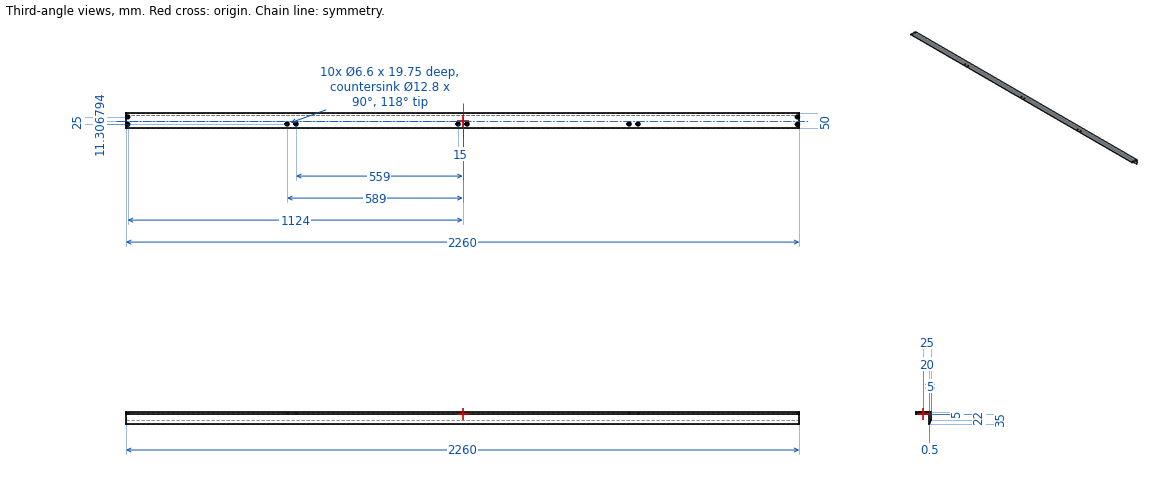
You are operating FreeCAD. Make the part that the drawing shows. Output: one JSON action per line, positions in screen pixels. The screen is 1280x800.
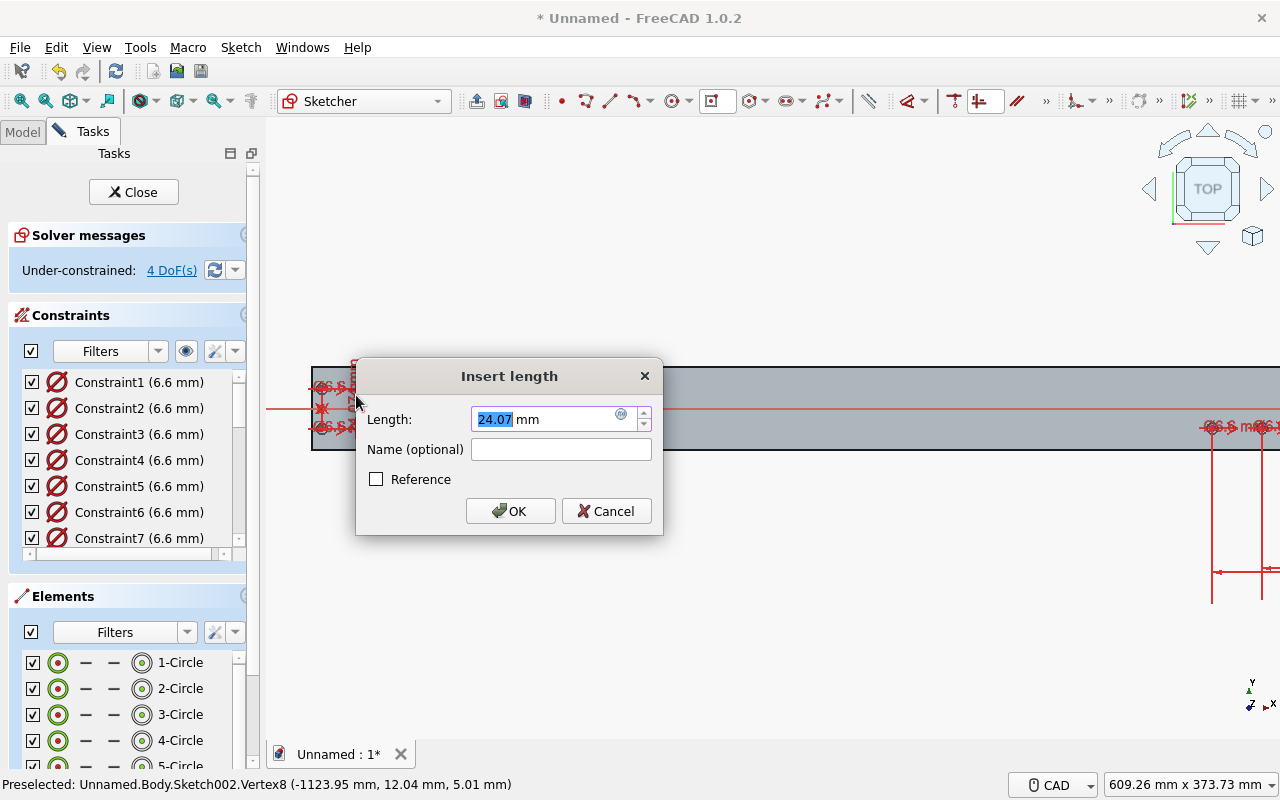
{"action": "type", "text": "25"}
{"action": "key", "text": "Return"}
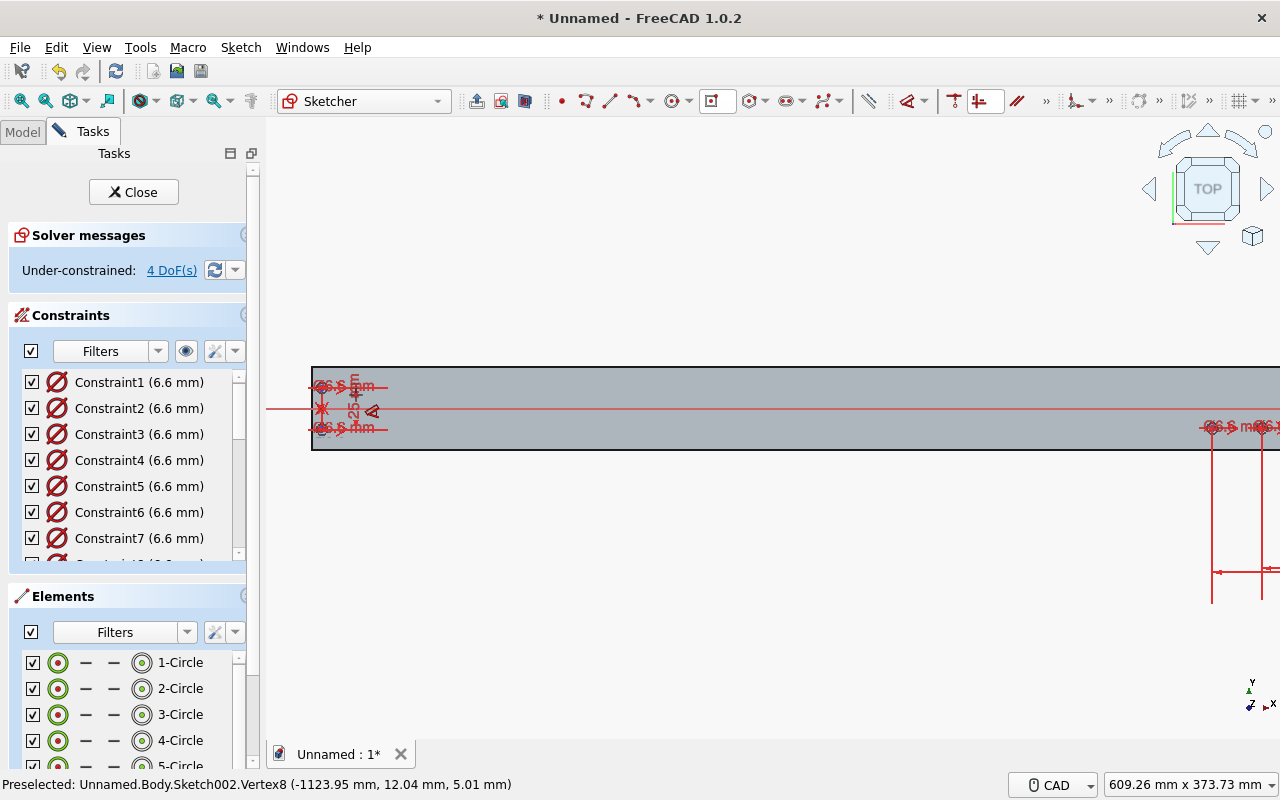
{"action": "scroll", "coordinate": [410, 432], "scroll_direction": "down", "scroll_amount": 9}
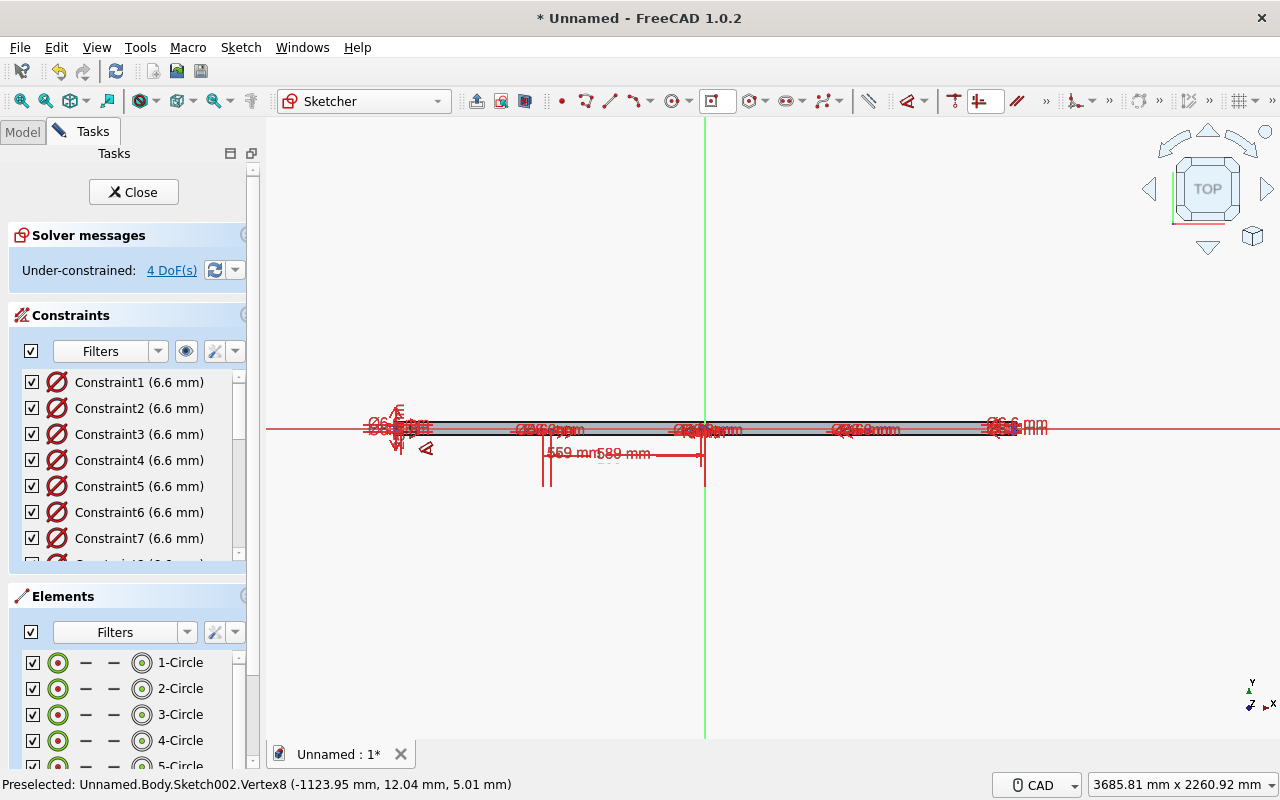
{"action": "scroll", "coordinate": [396, 432], "scroll_direction": "up", "scroll_amount": 3}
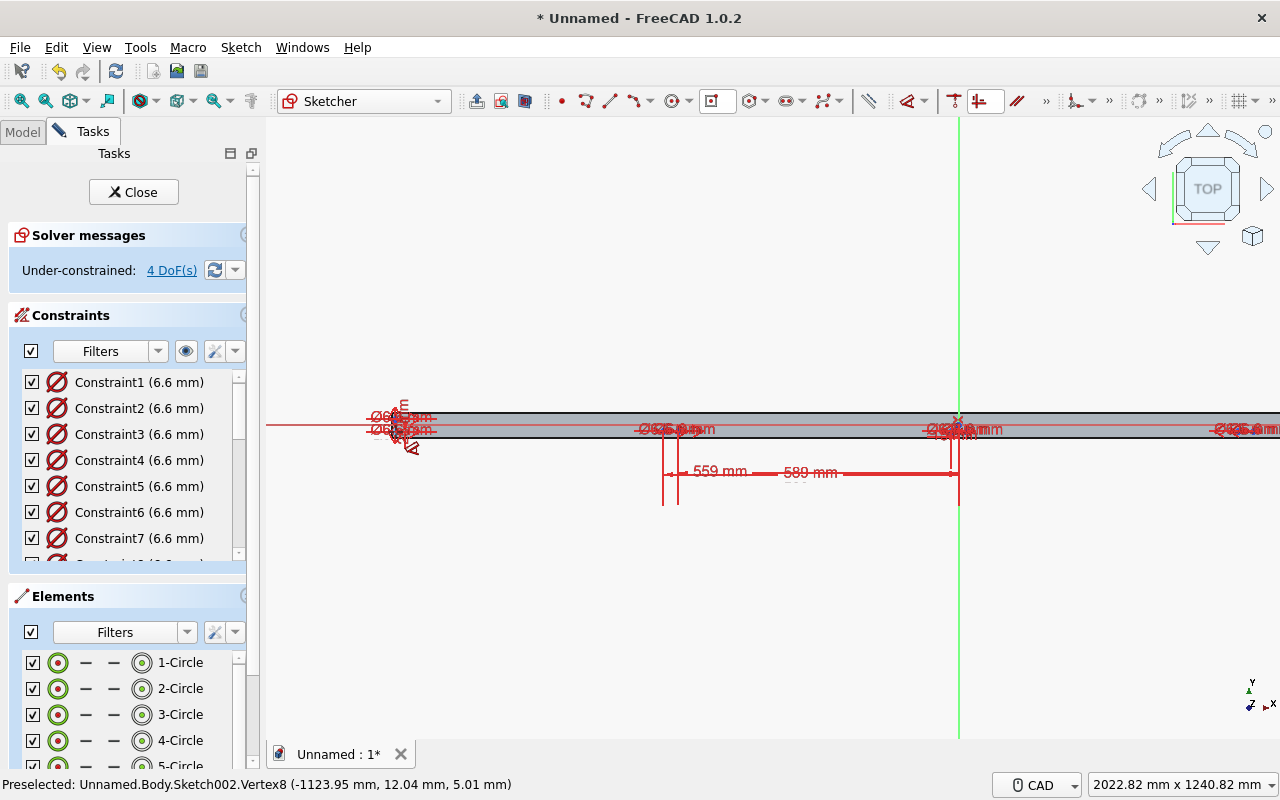
{"action": "left_click", "coordinate": [395, 432]}
{"action": "left_click", "coordinate": [547, 466]}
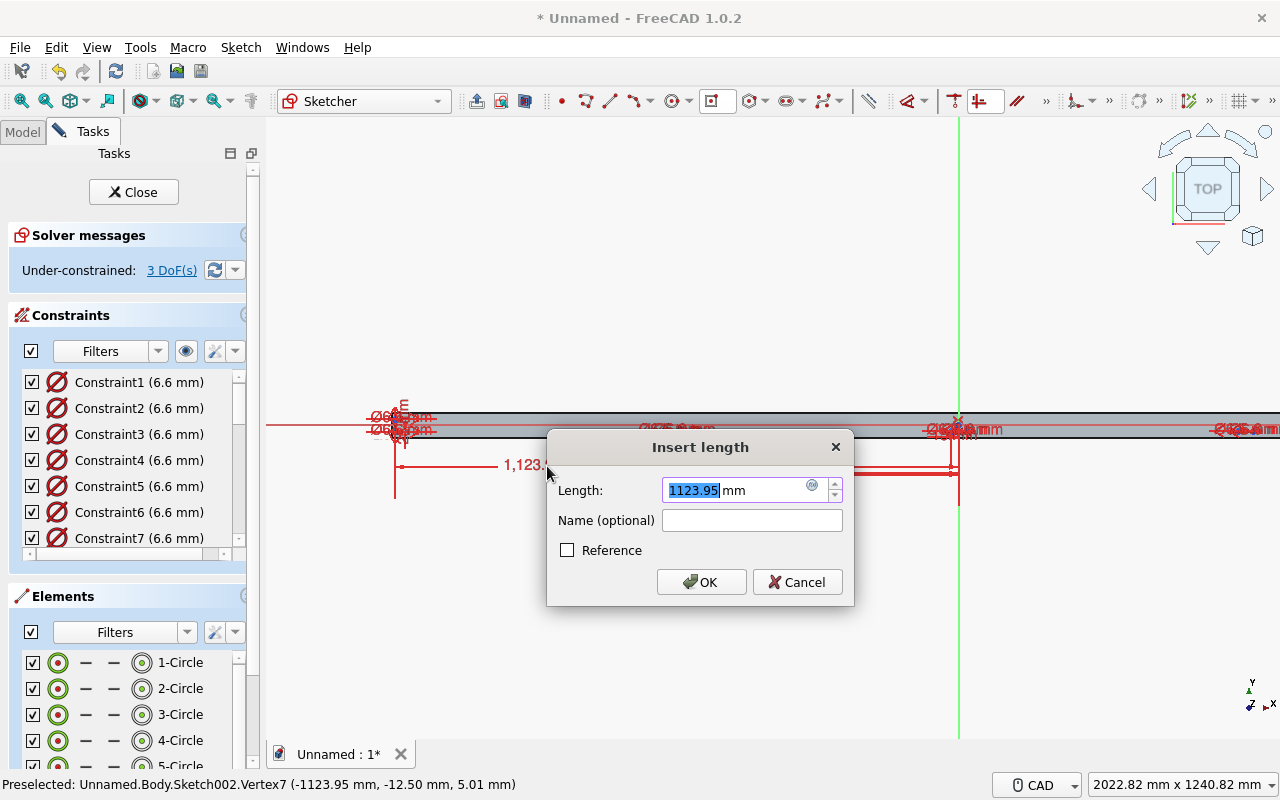
{"action": "type", "text": "1124"}
{"action": "key", "text": "Return"}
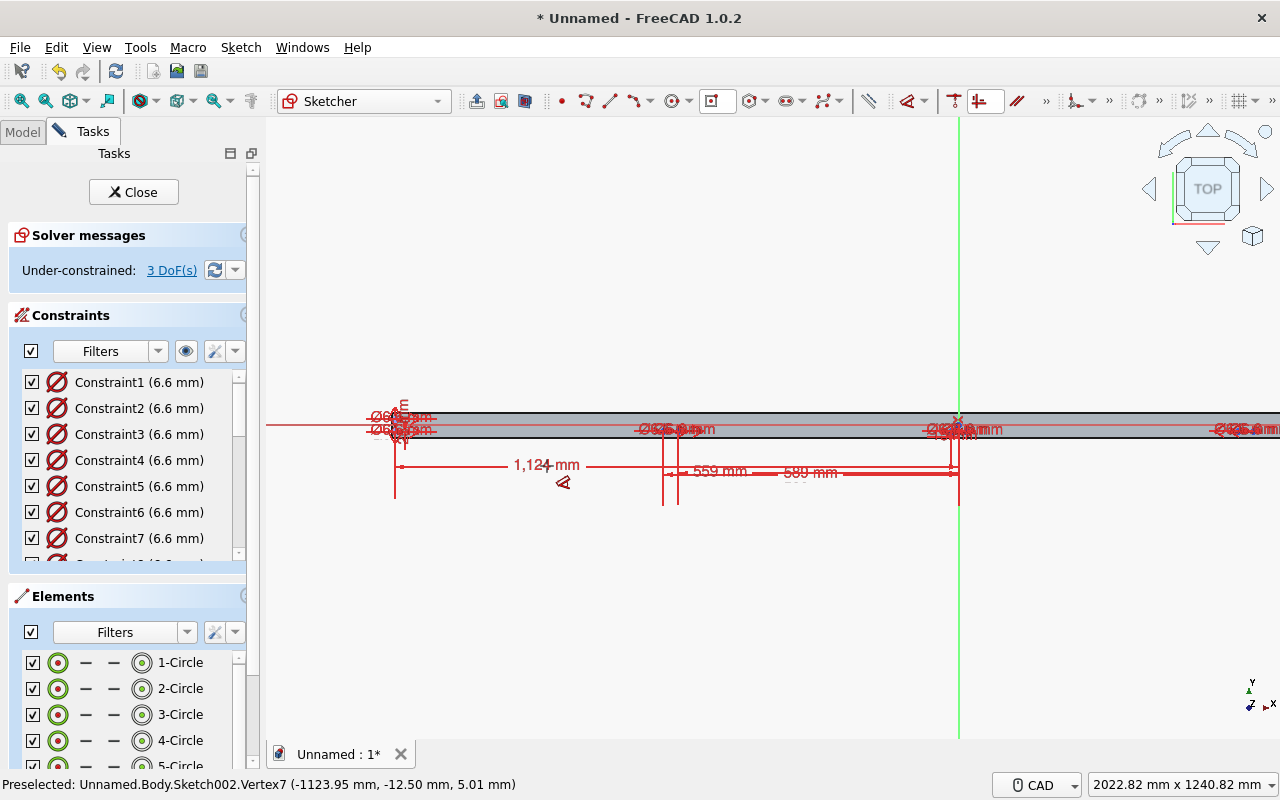
{"action": "scroll", "coordinate": [663, 431], "scroll_direction": "up", "scroll_amount": 10}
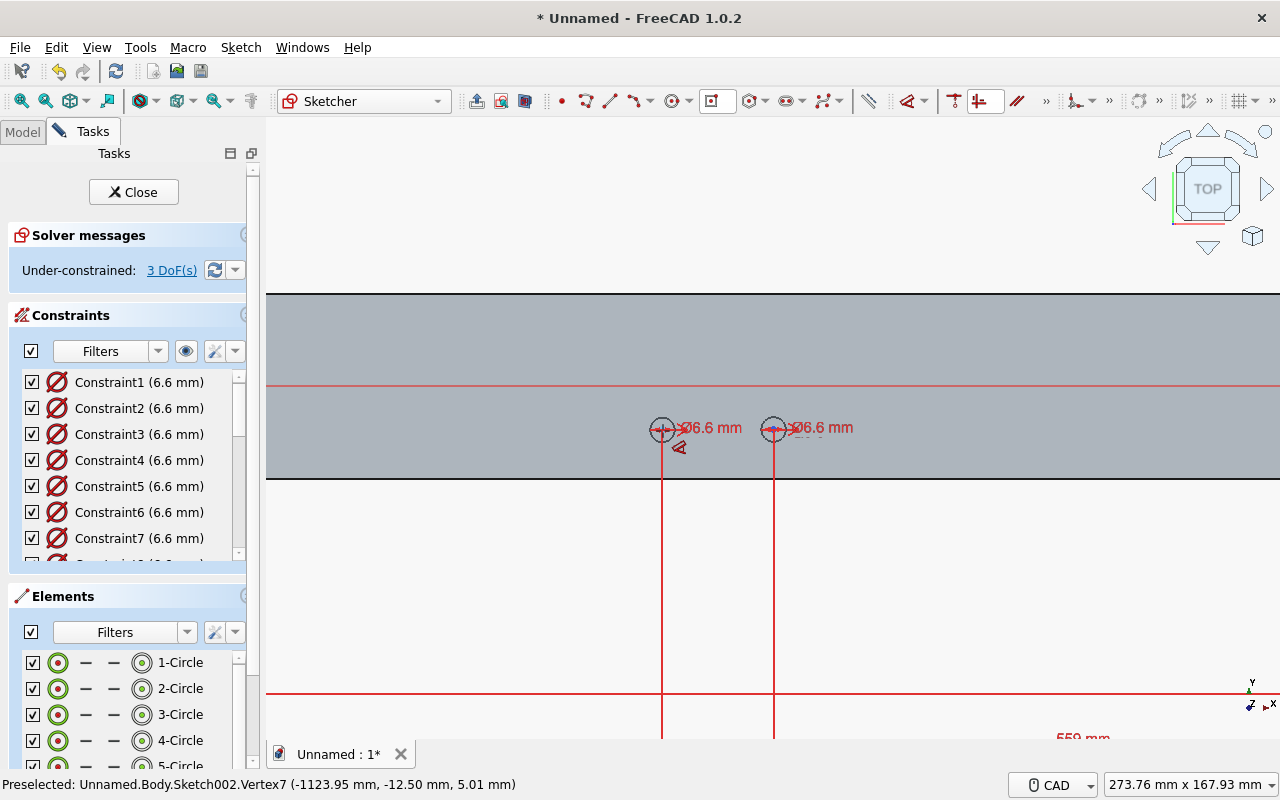
{"action": "left_click", "coordinate": [662, 430]}
{"action": "left_click", "coordinate": [628, 408]}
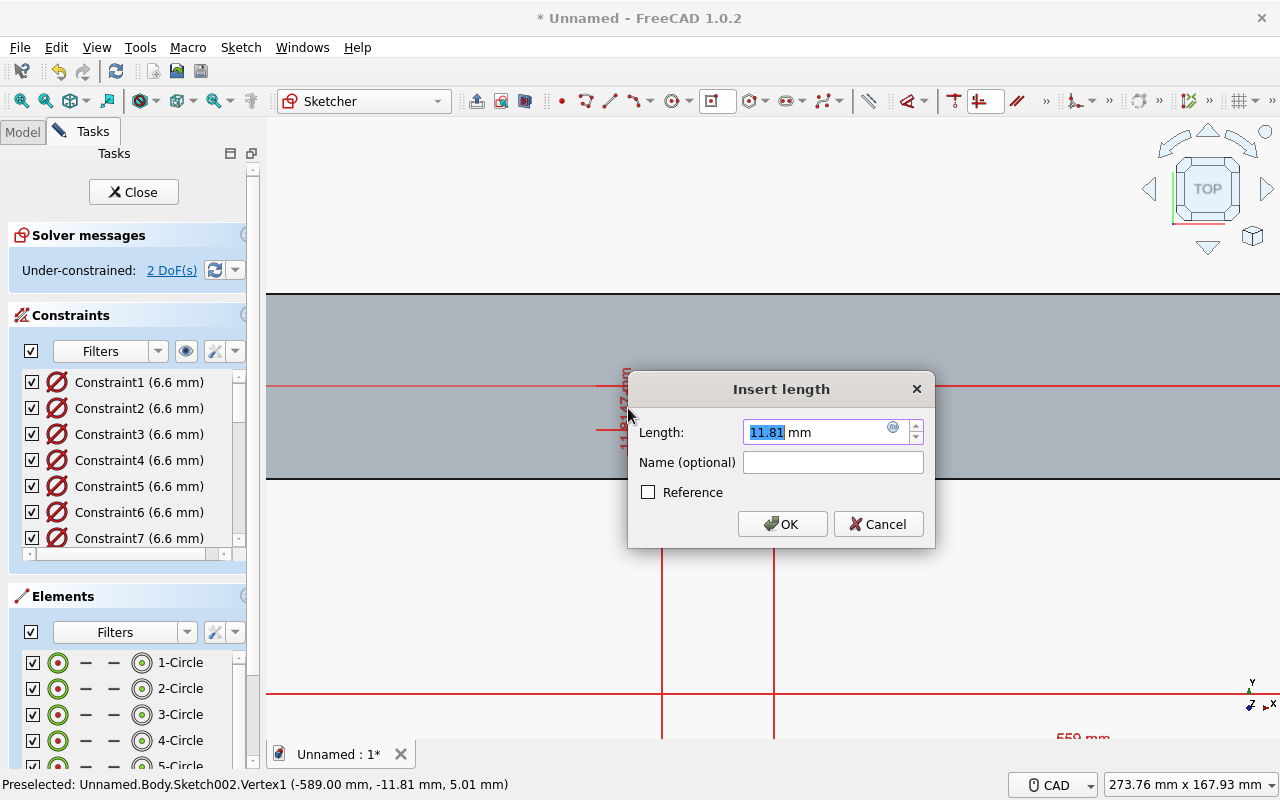
{"action": "type", "text": "11.306794"}
{"action": "key", "text": "Return"}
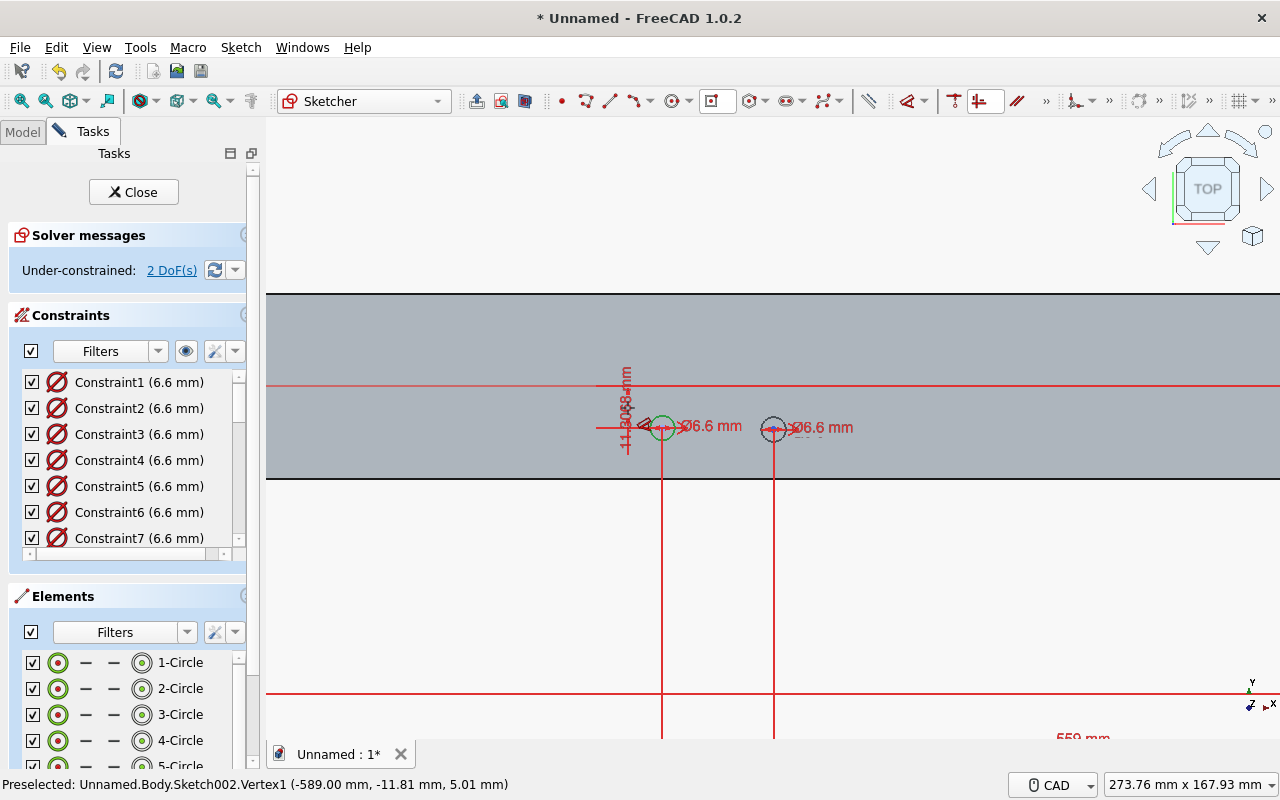
{"action": "left_click", "coordinate": [774, 430]}
{"action": "left_click", "coordinate": [740, 408]}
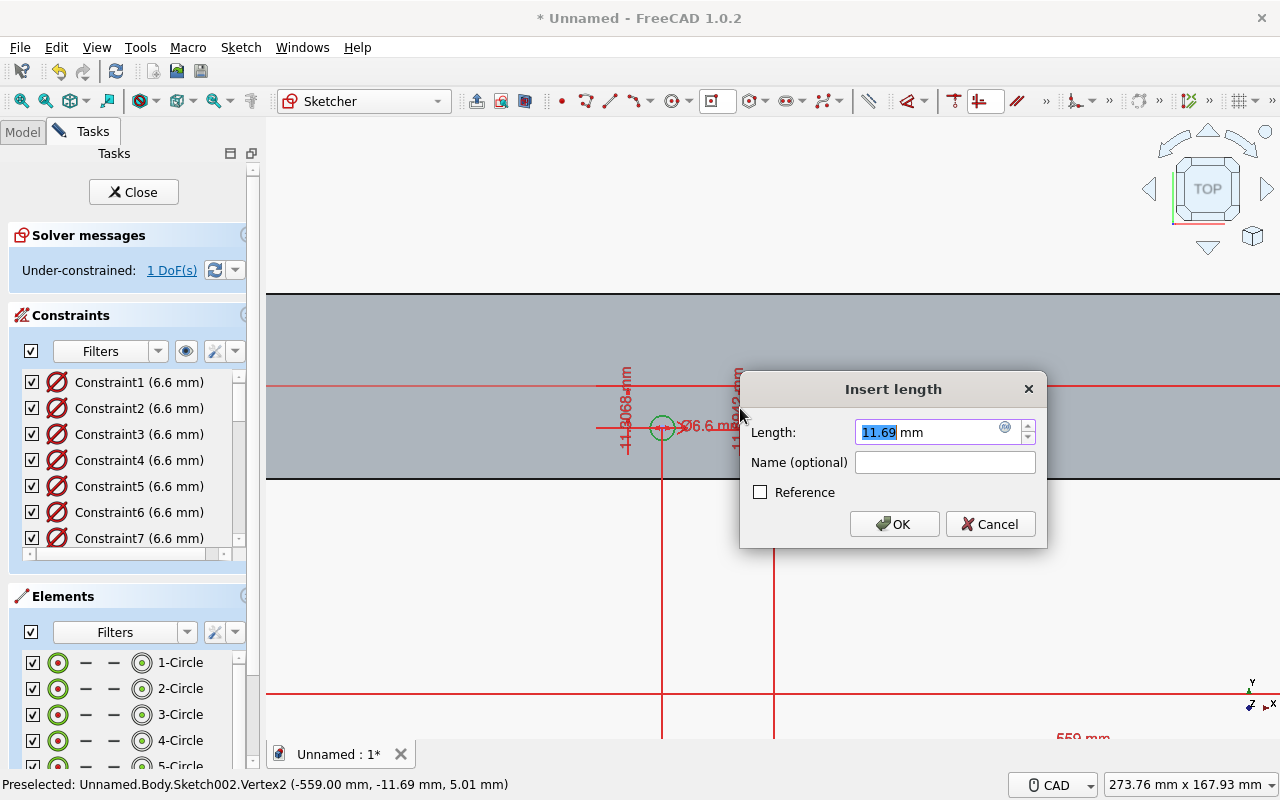
{"action": "type", "text": "11.306794"}
{"action": "key", "text": "Return"}